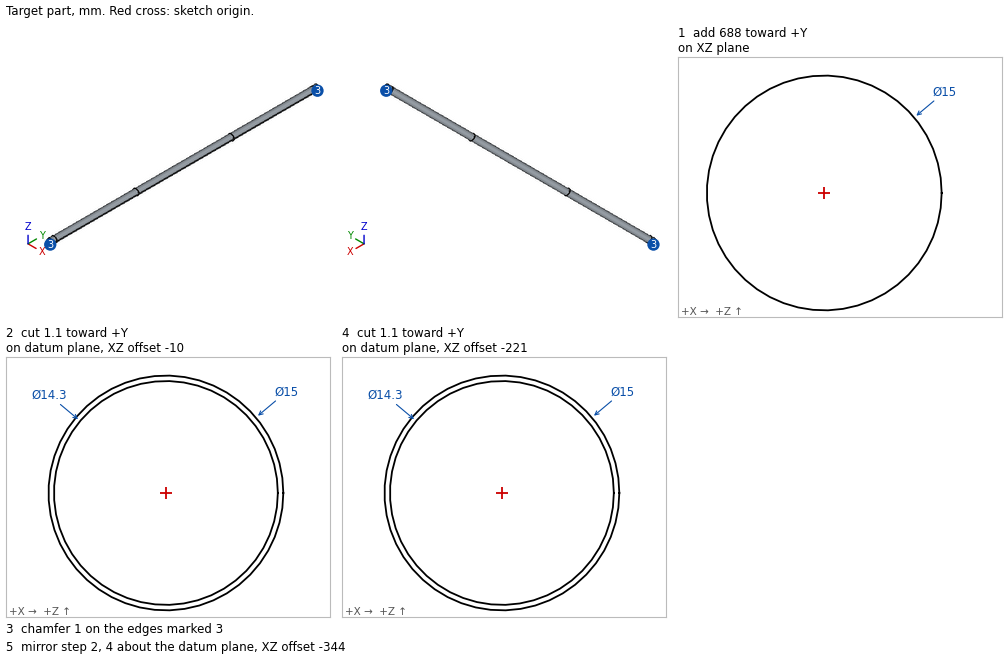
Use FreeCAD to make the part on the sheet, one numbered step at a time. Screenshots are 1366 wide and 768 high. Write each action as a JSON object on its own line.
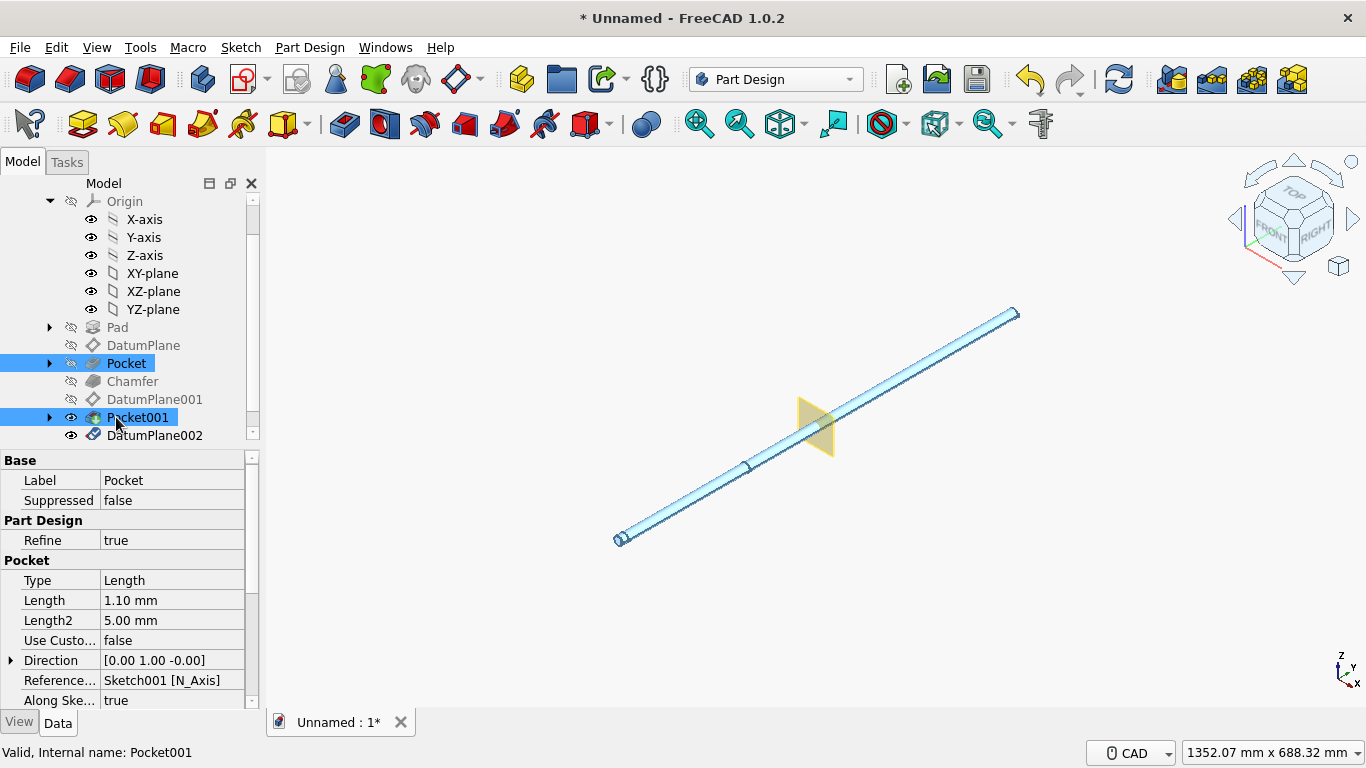
{"action": "left_click", "coordinate": [1172, 80]}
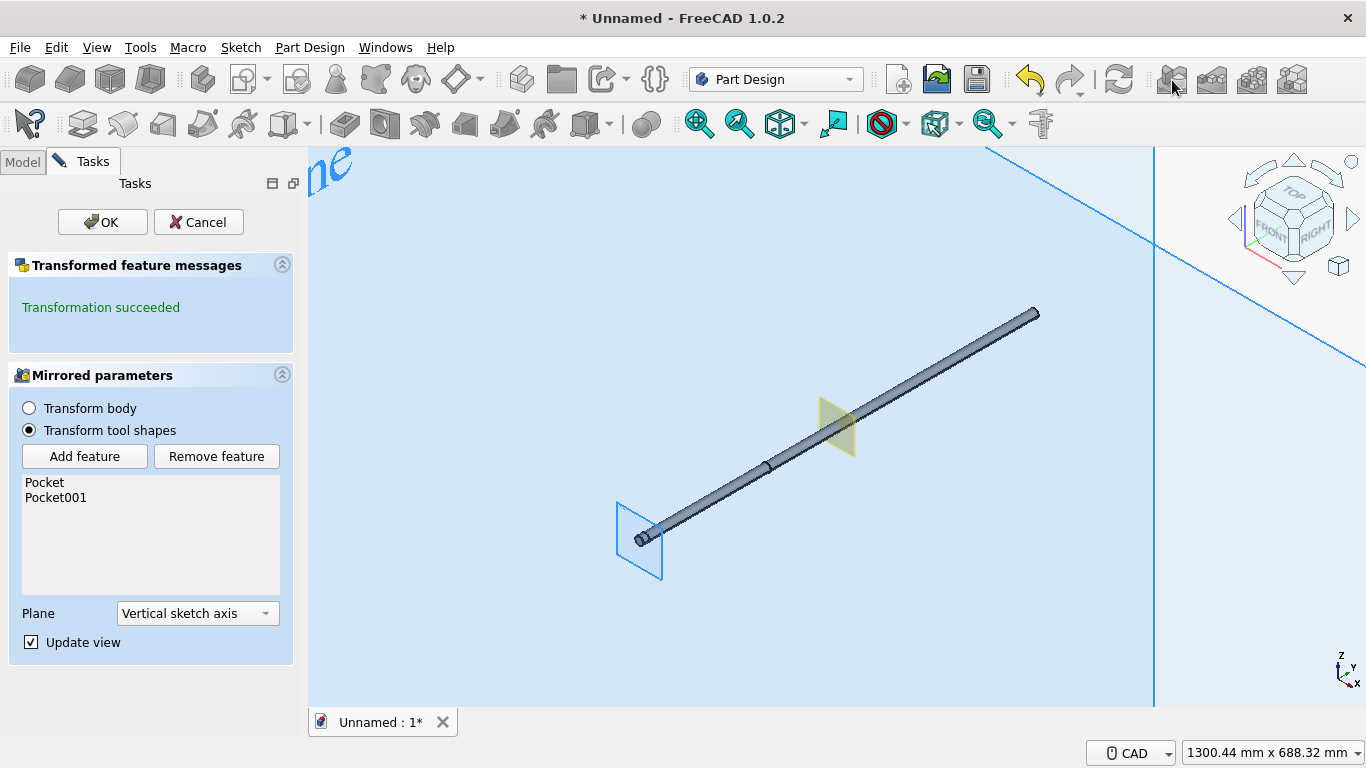
{"action": "left_click", "coordinate": [198, 614]}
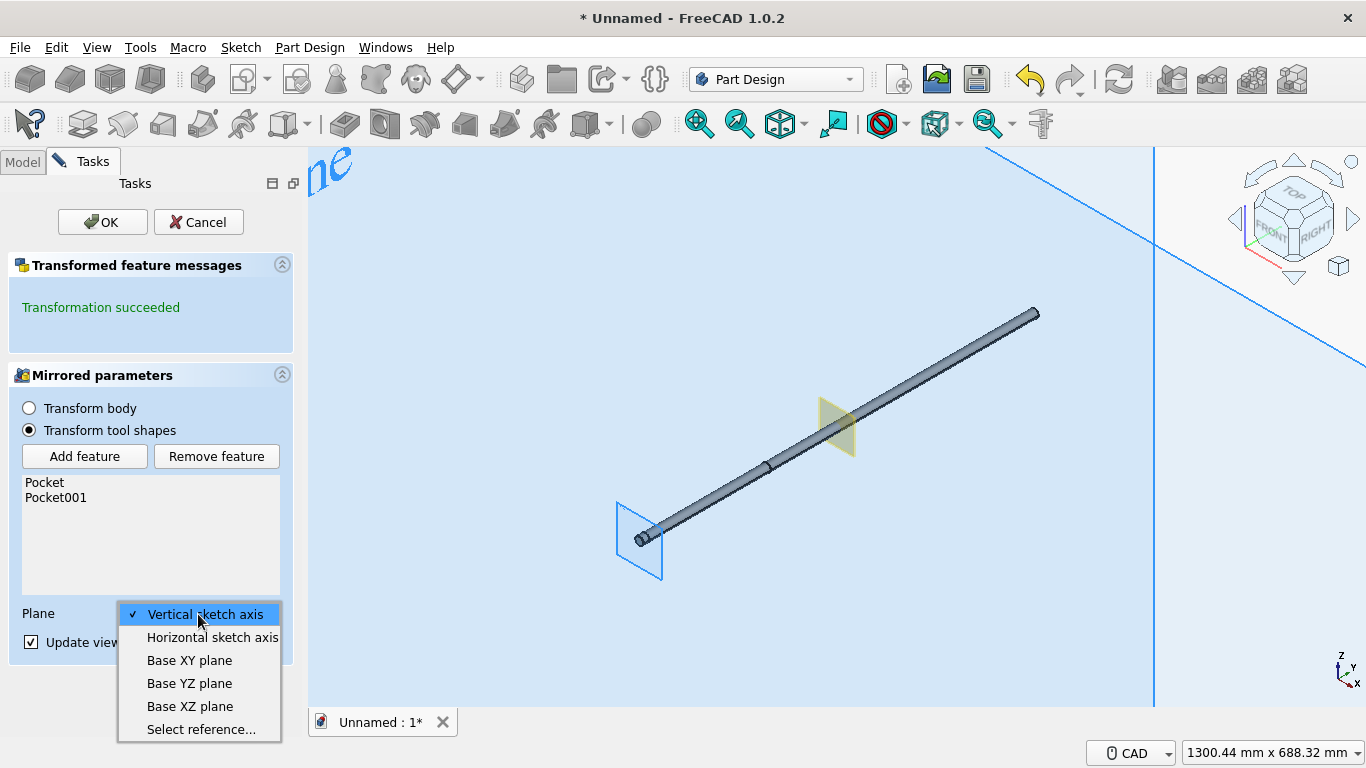
{"action": "left_click", "coordinate": [198, 730]}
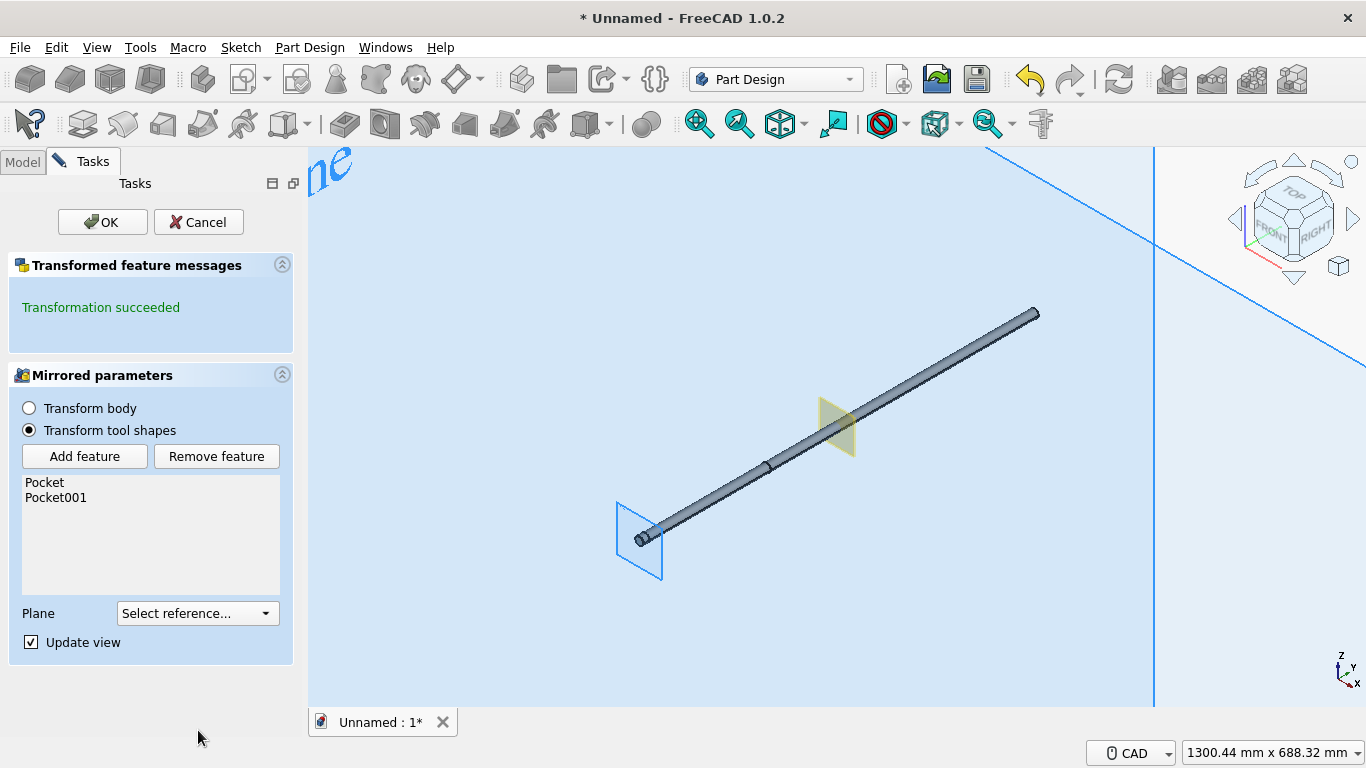
{"action": "left_click", "coordinate": [23, 161]}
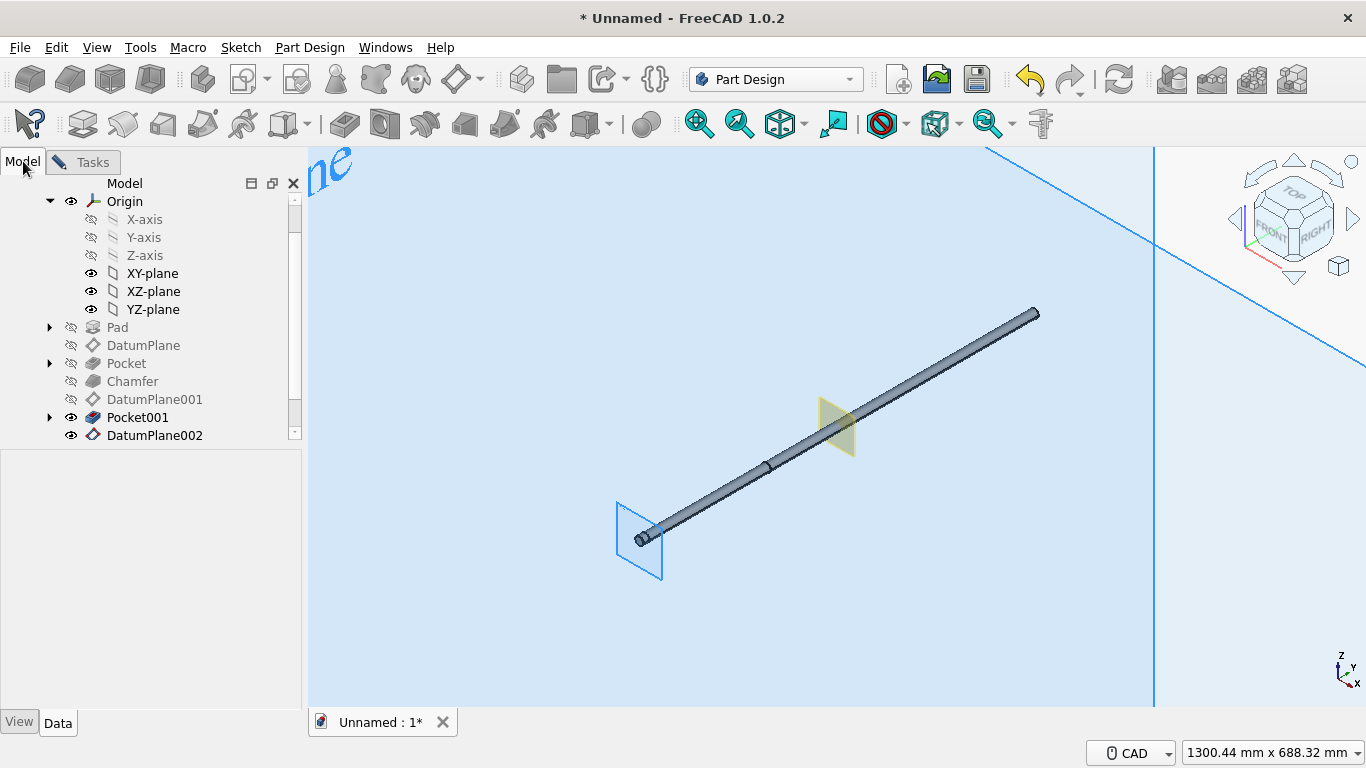
{"action": "left_click", "coordinate": [116, 435]}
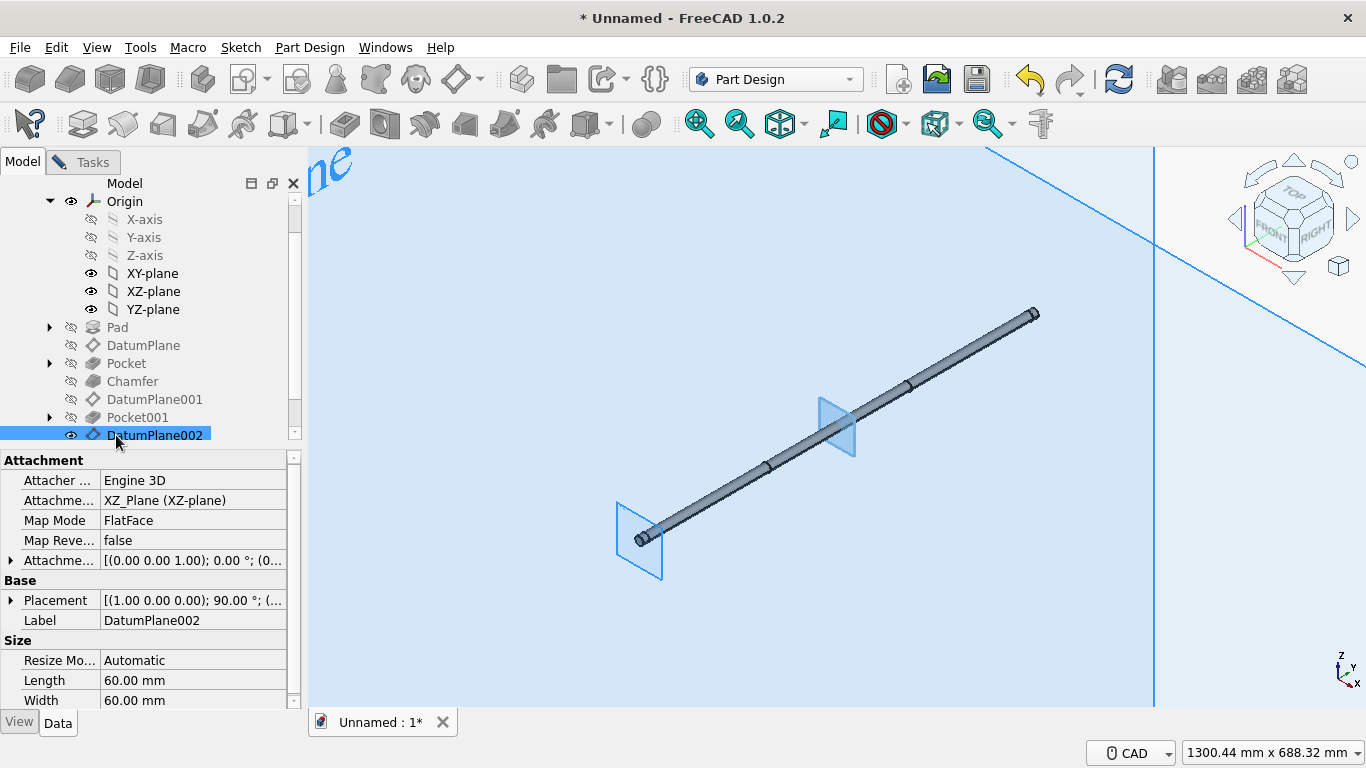
{"action": "left_click", "coordinate": [84, 161]}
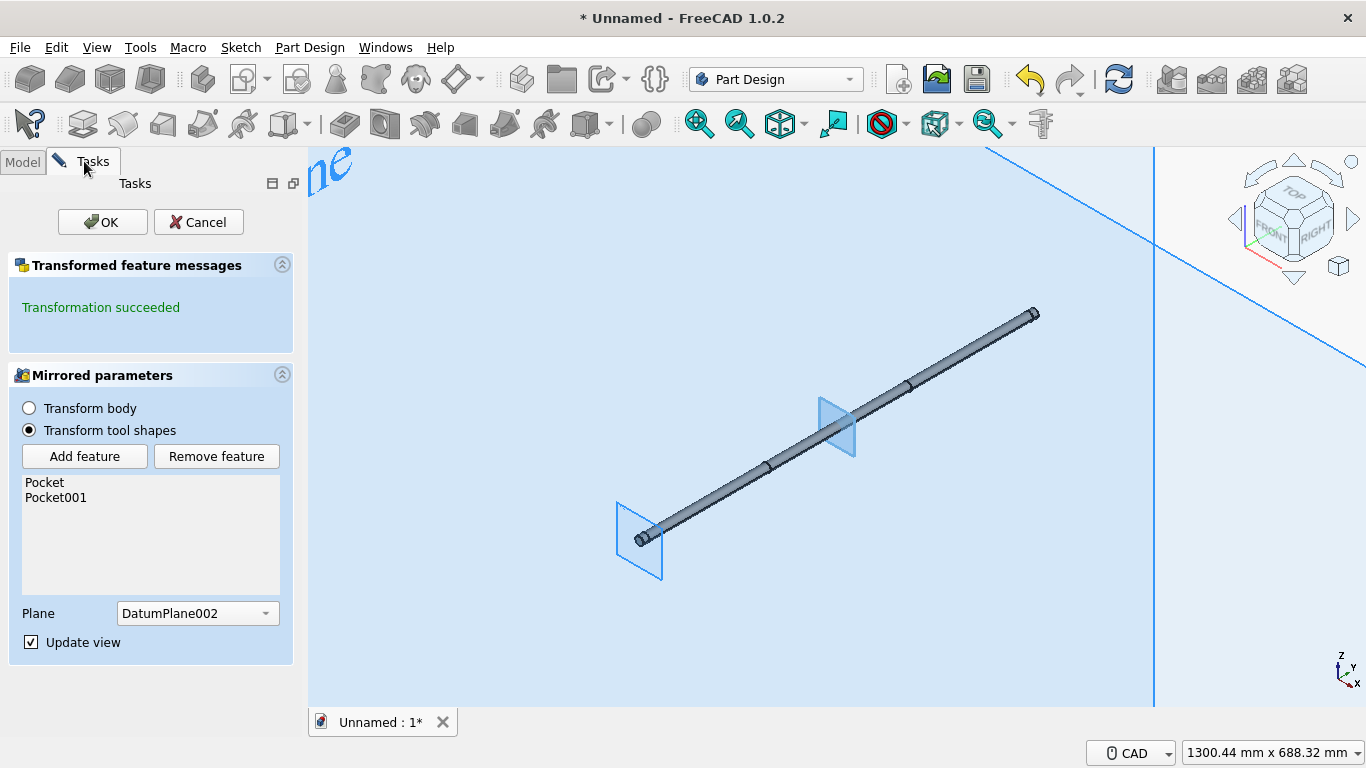
{"action": "left_click", "coordinate": [103, 222]}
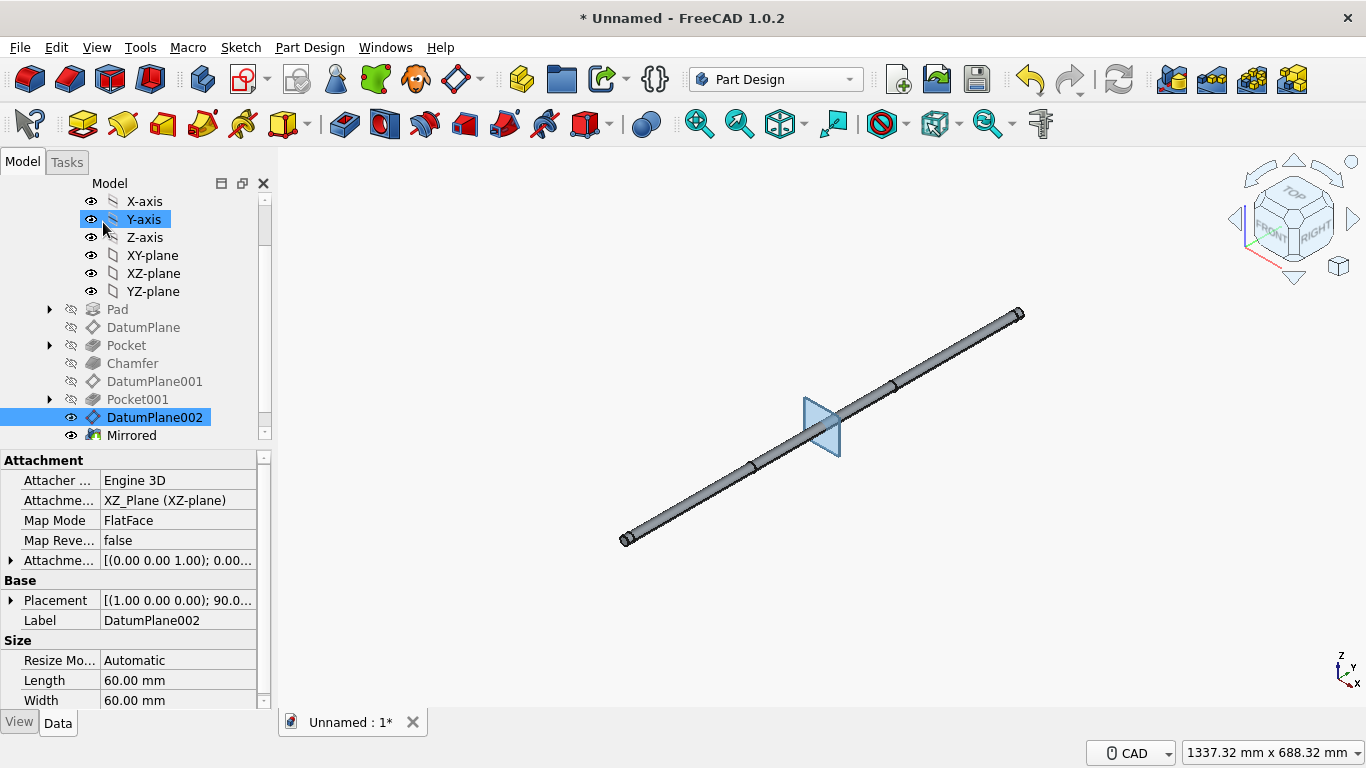
{"action": "left_click", "coordinate": [116, 417]}
{"action": "key", "text": "space"}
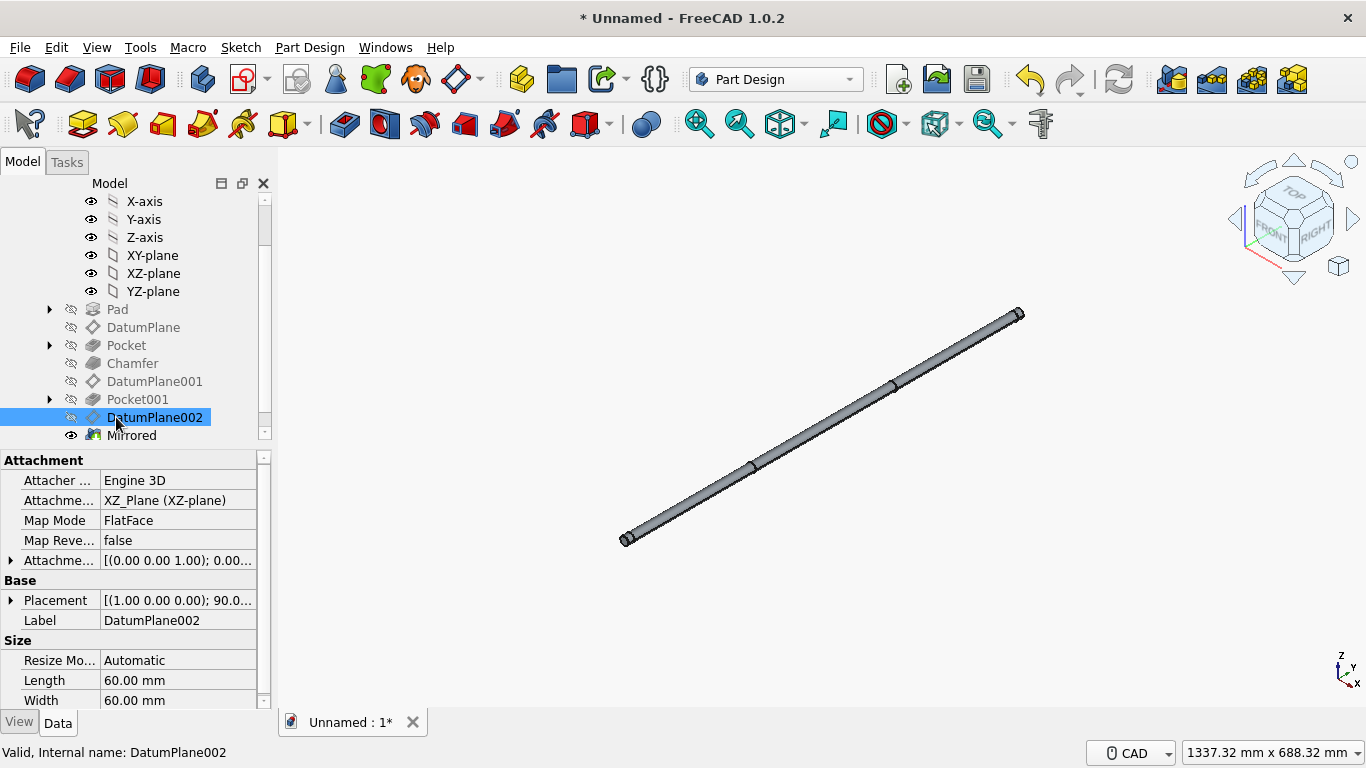
{"action": "left_click", "coordinate": [700, 124]}